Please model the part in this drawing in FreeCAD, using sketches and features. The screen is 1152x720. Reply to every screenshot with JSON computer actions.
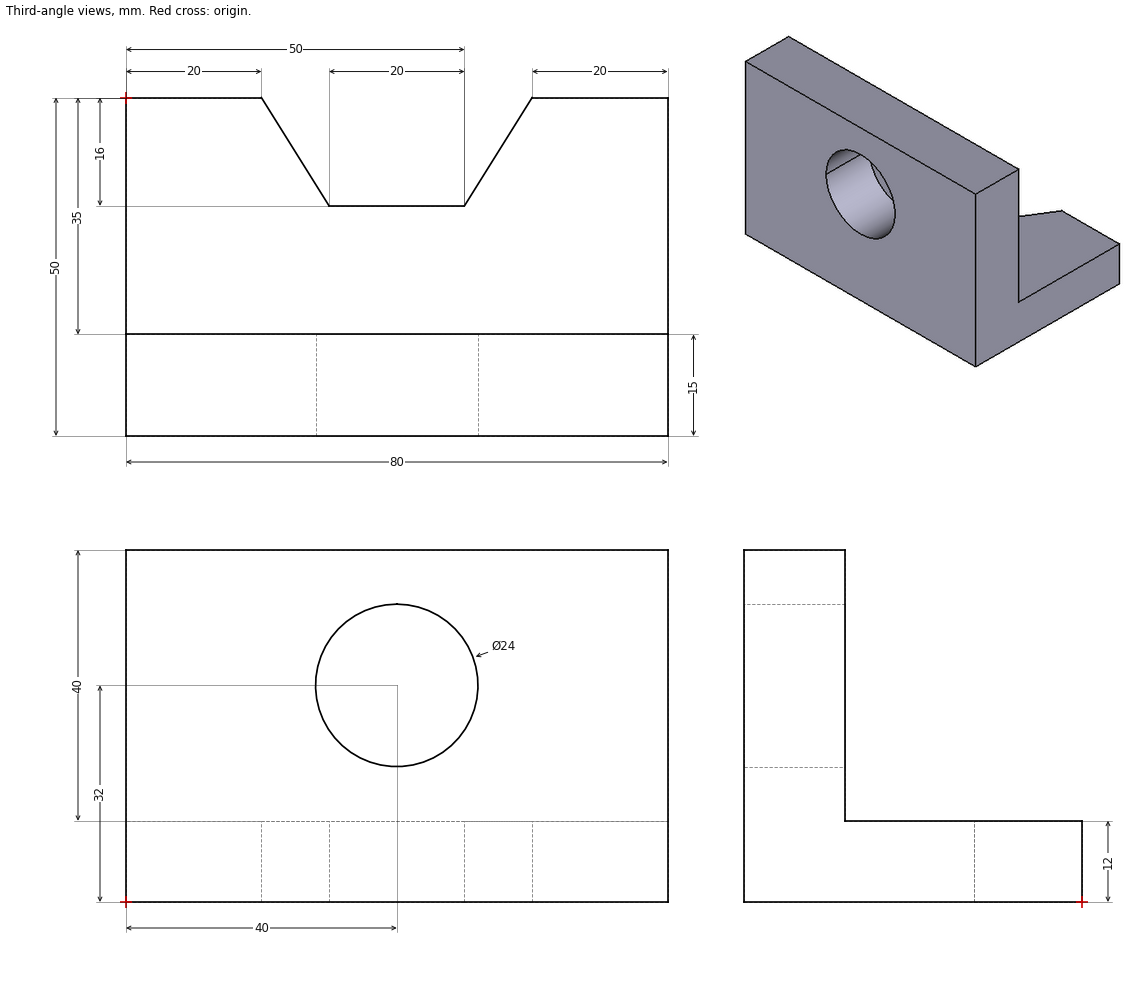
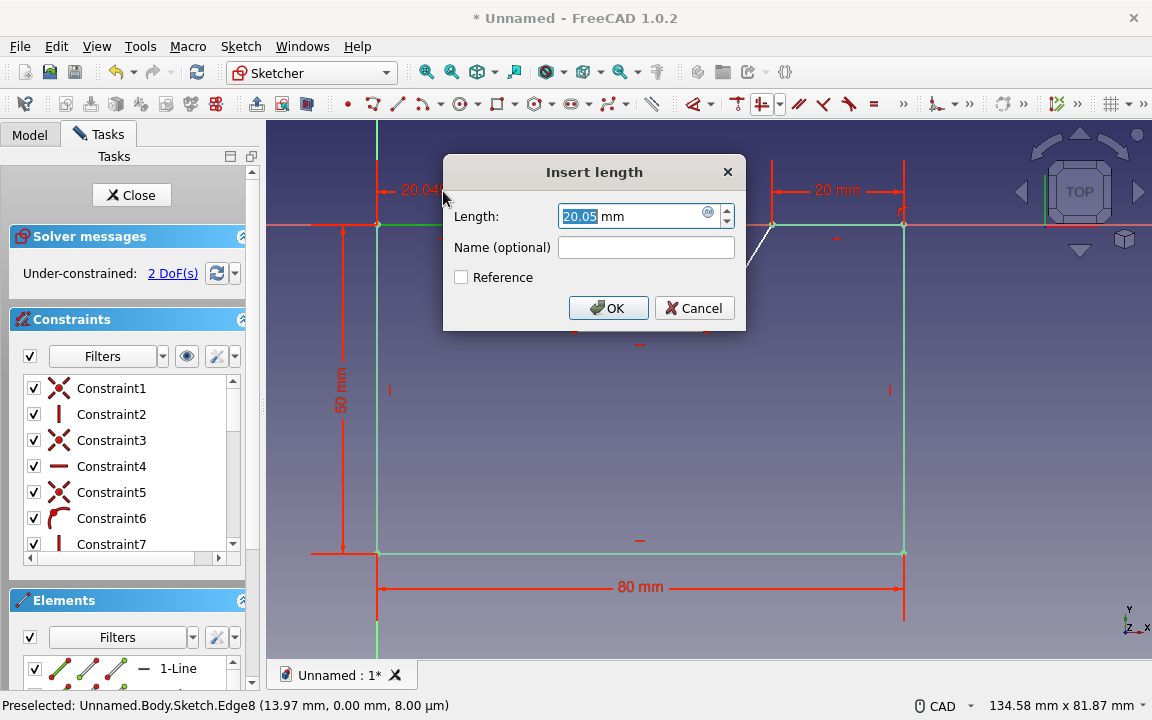
{"action": "type", "text": "20"}
{"action": "key", "text": "Return"}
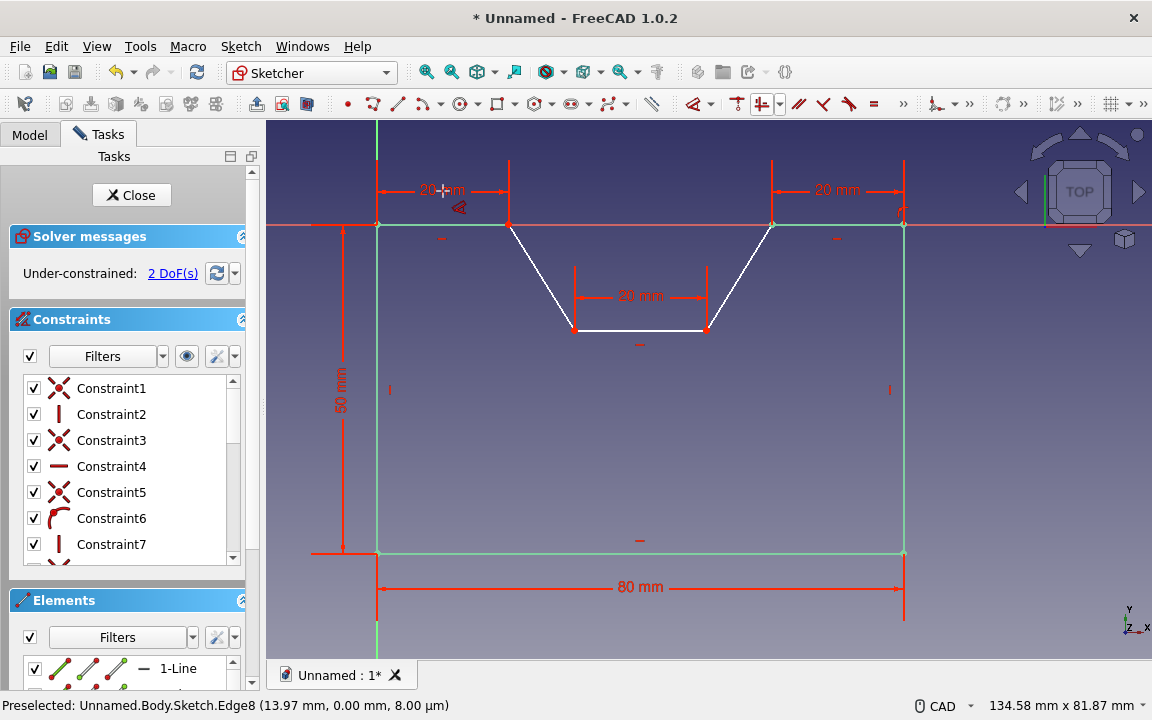
{"action": "left_click", "coordinate": [707, 331]}
{"action": "left_click", "coordinate": [542, 191]}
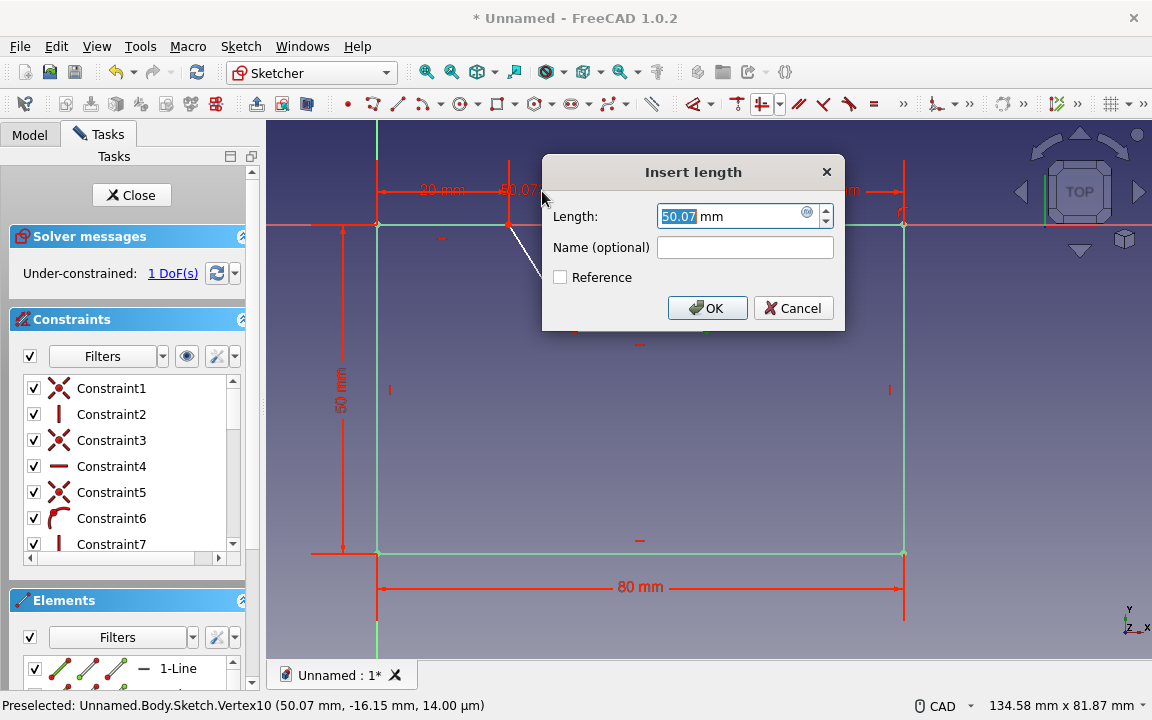
{"action": "type", "text": "50"}
{"action": "key", "text": "Return"}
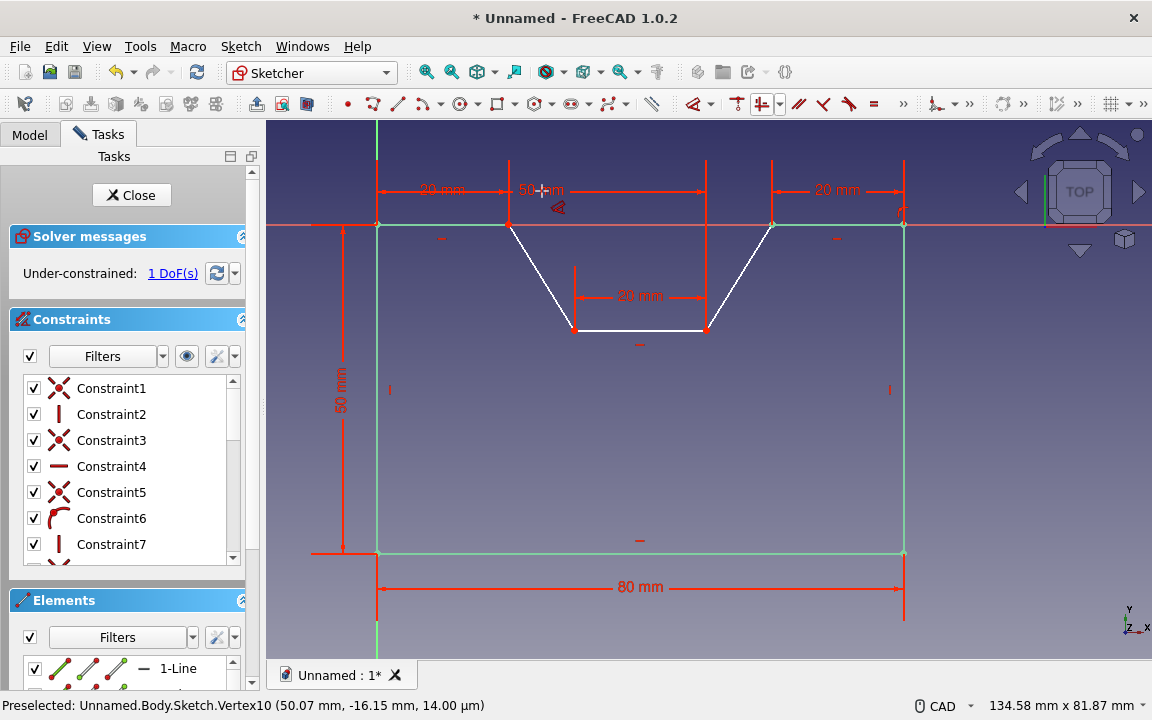
{"action": "left_click", "coordinate": [706, 331]}
{"action": "left_click", "coordinate": [343, 278]}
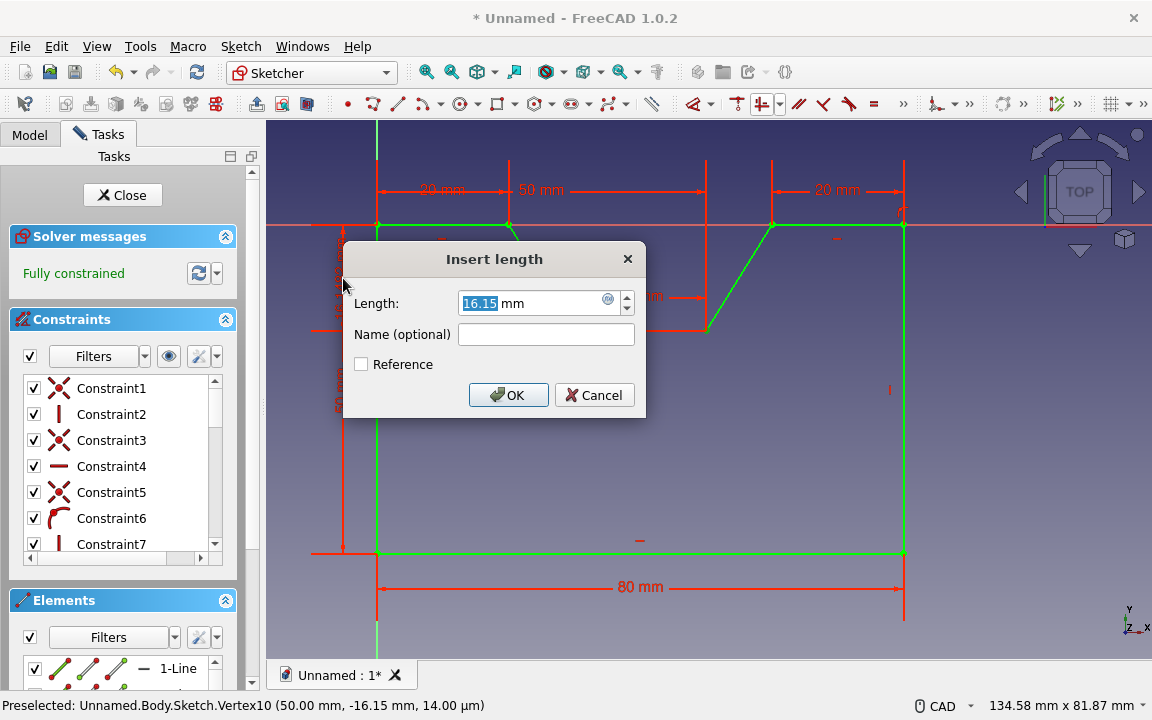
{"action": "type", "text": "16"}
{"action": "key", "text": "Return"}
{"action": "key", "text": "Escape"}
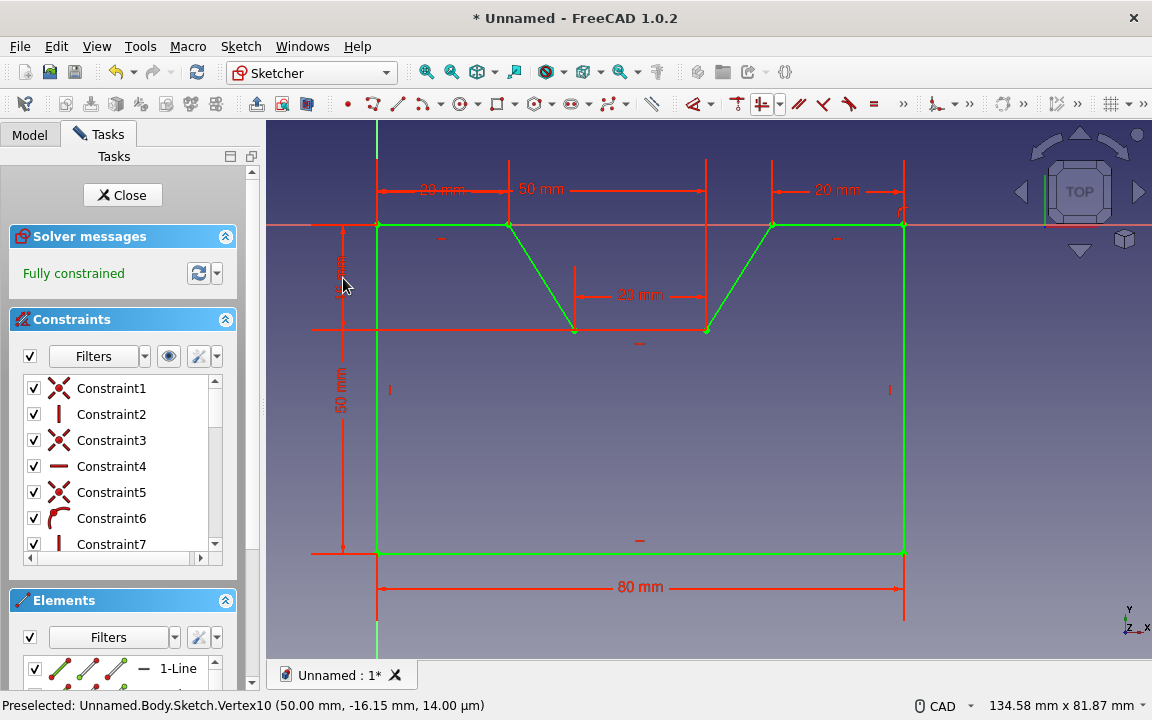
{"action": "left_click", "coordinate": [123, 195]}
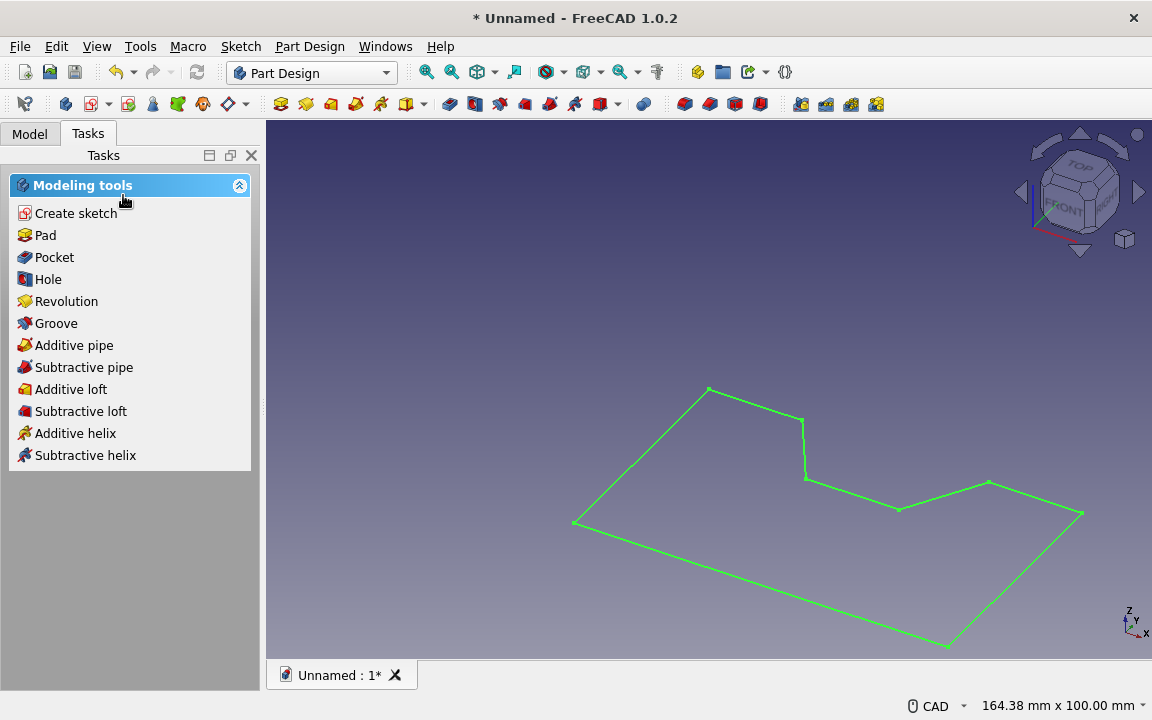
{"action": "left_click", "coordinate": [281, 104]}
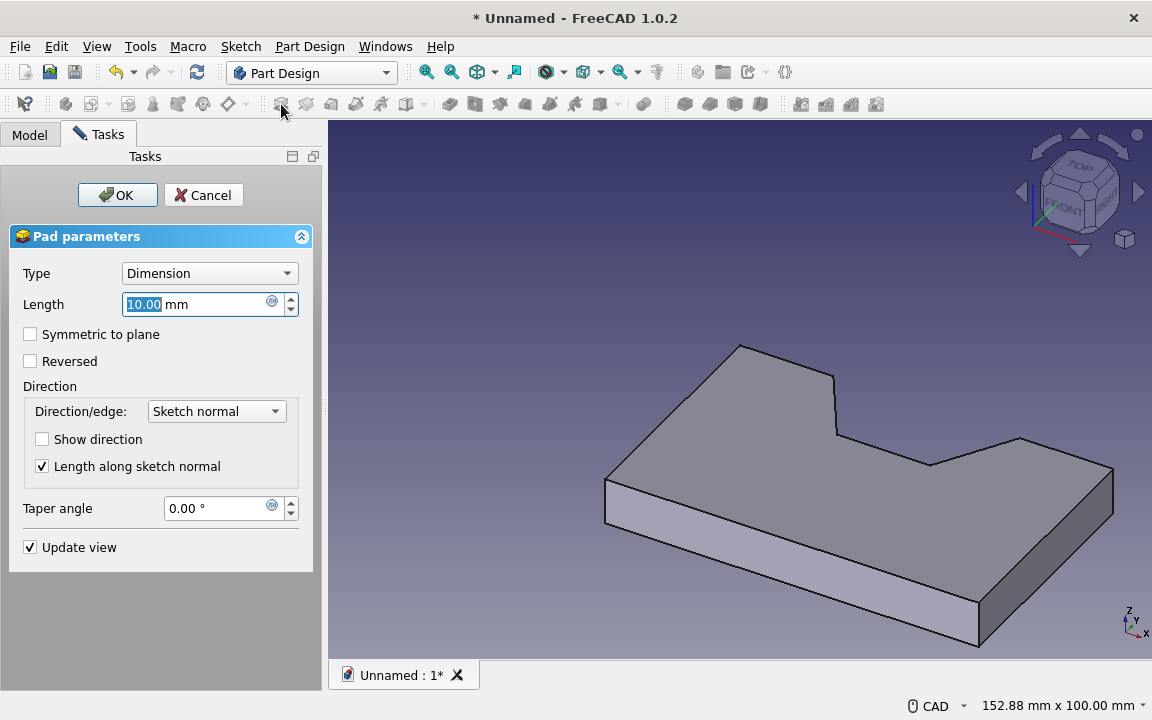
{"action": "type", "text": "12"}
{"action": "key", "text": "Tab"}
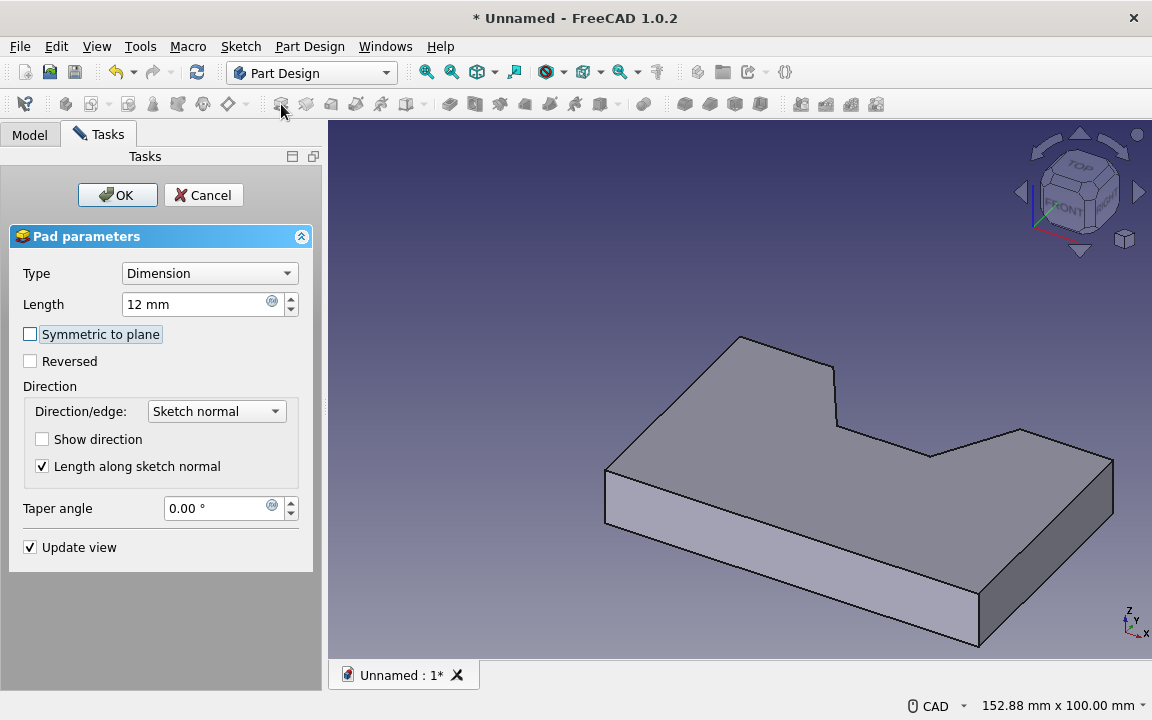
{"action": "left_click", "coordinate": [118, 195]}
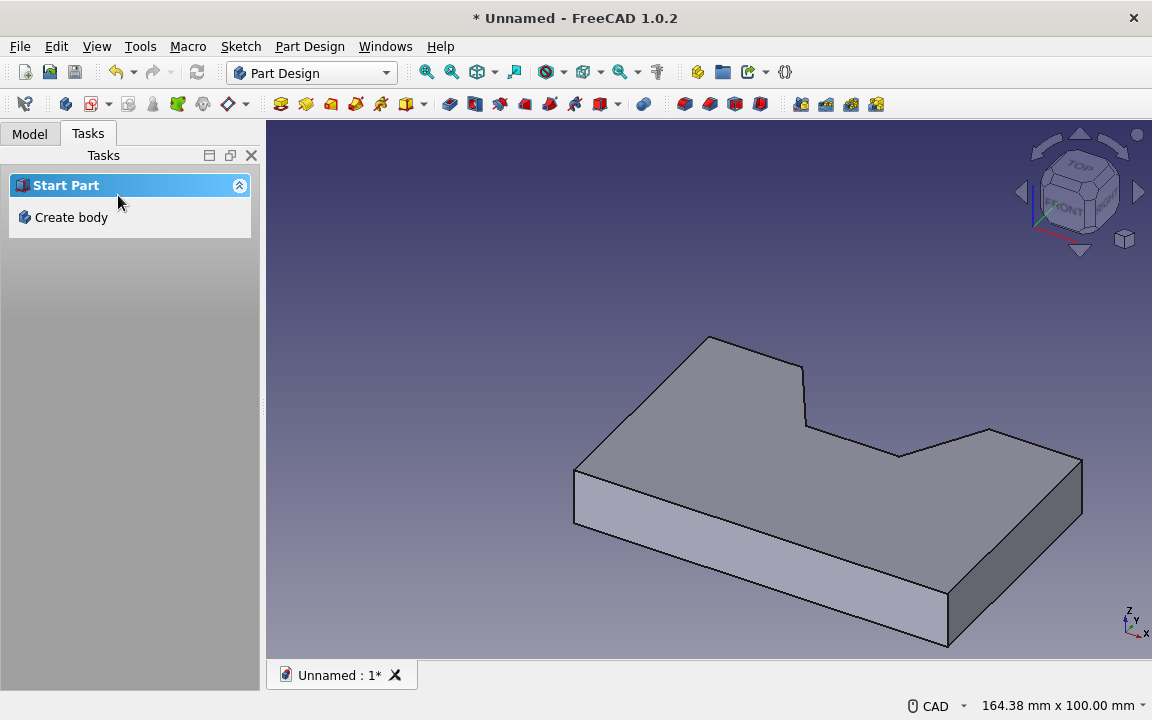
{"action": "left_click", "coordinate": [916, 519]}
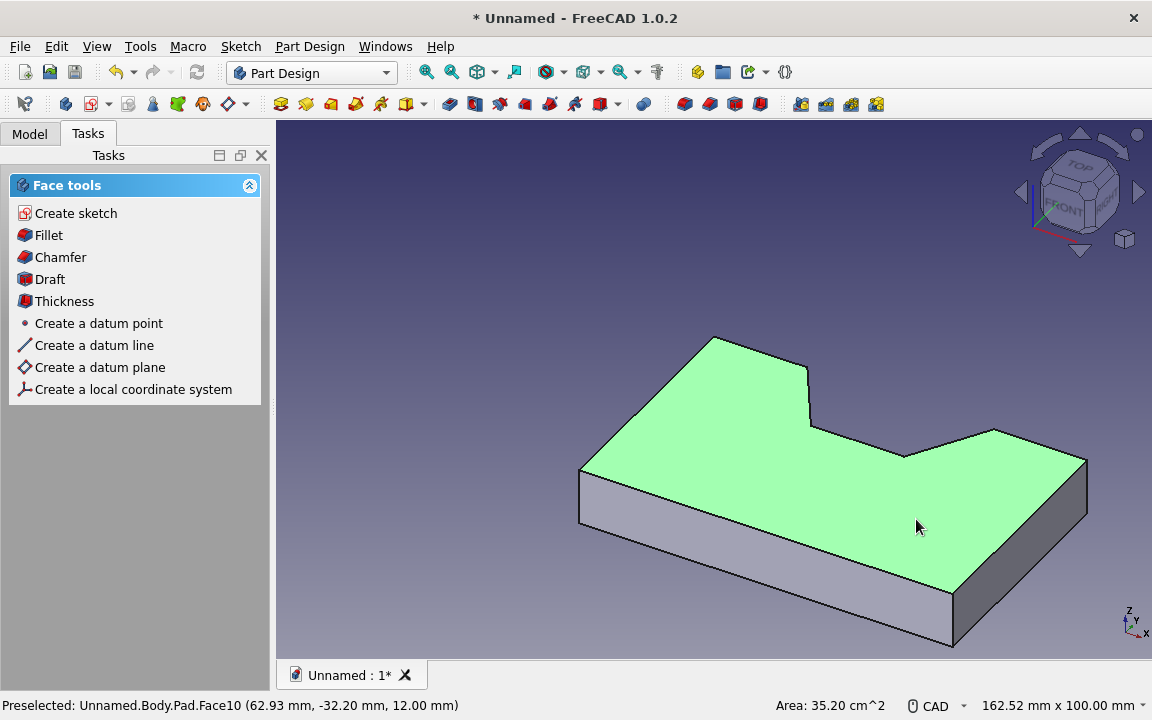
{"action": "left_click", "coordinate": [90, 104]}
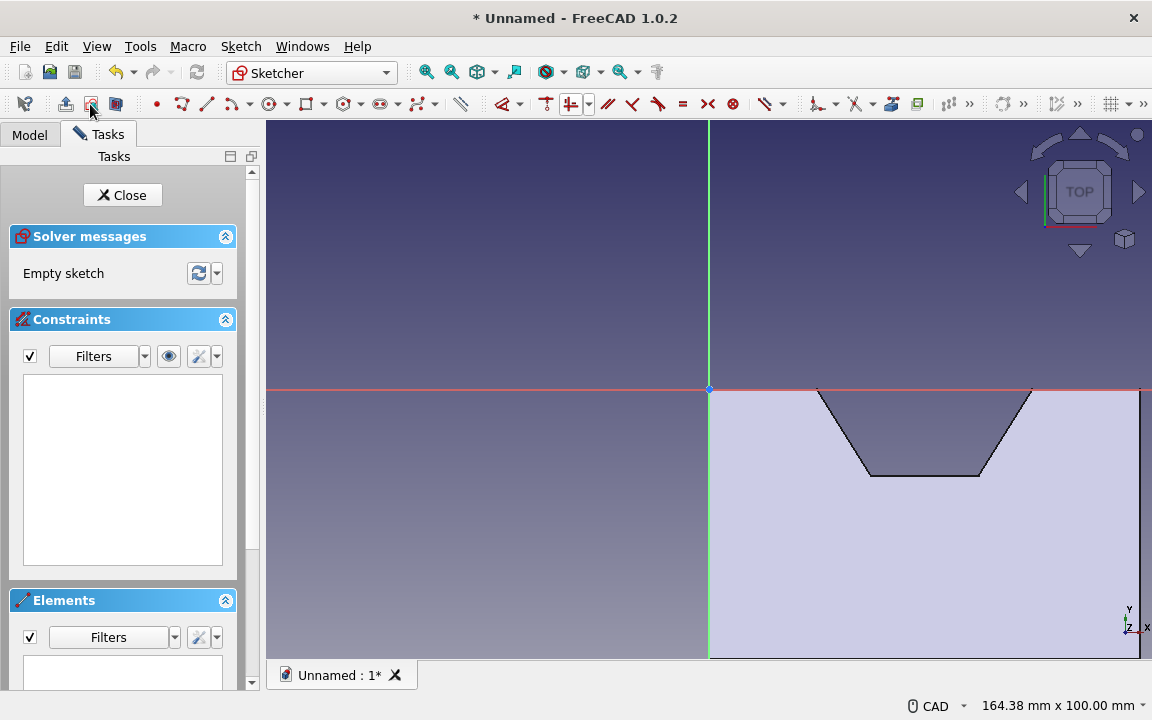
{"action": "scroll", "coordinate": [294, 148], "scroll_direction": "down", "scroll_amount": 2}